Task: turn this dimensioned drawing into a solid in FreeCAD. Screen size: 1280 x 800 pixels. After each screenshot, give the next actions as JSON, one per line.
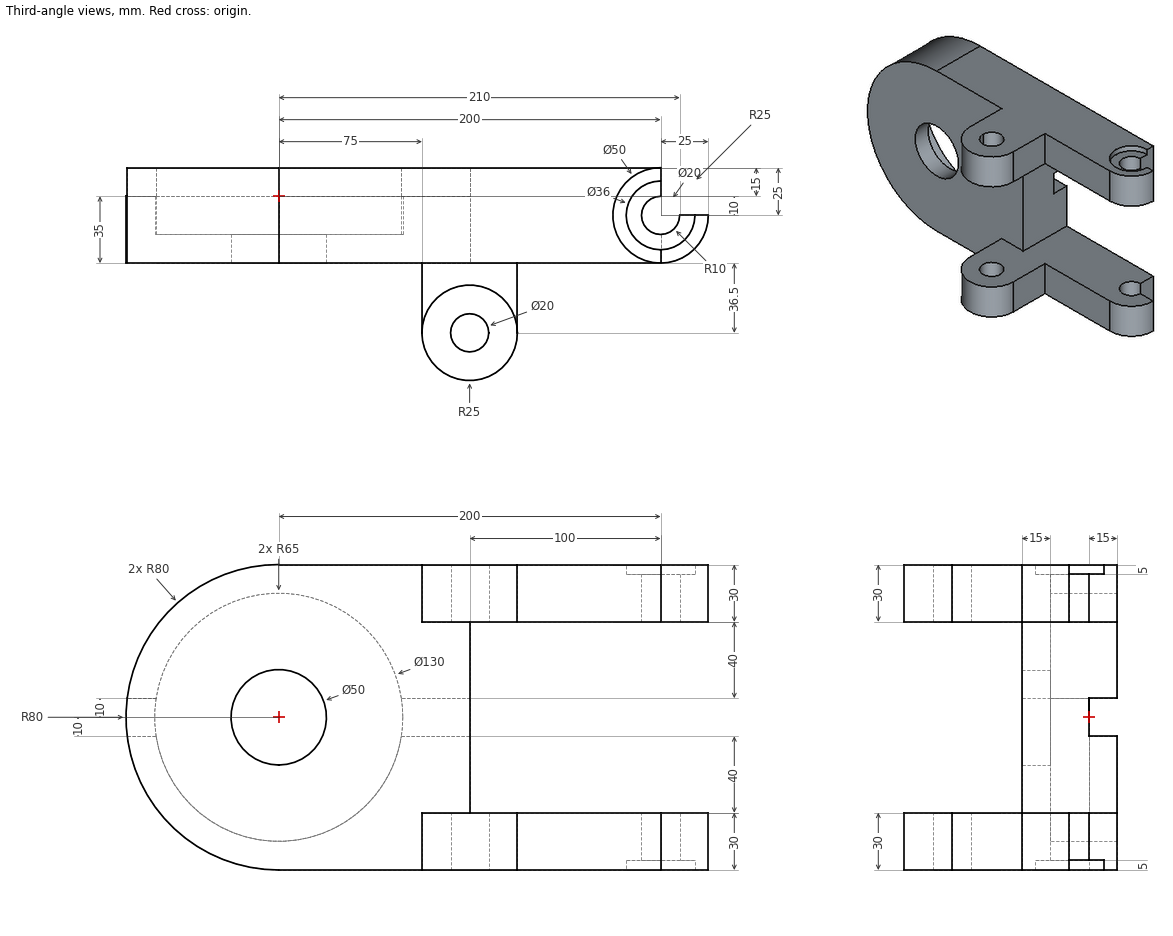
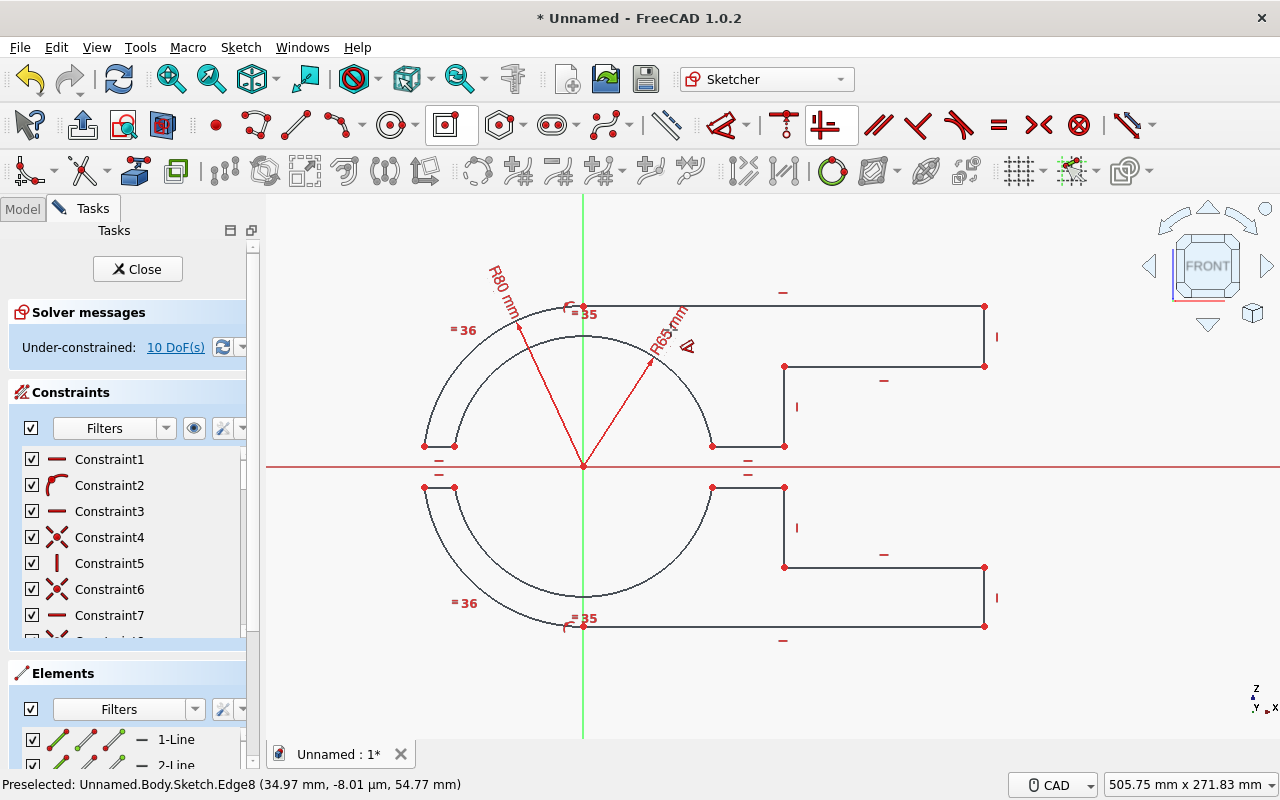
{"action": "left_click", "coordinate": [984, 324]}
{"action": "left_click", "coordinate": [1018, 337]}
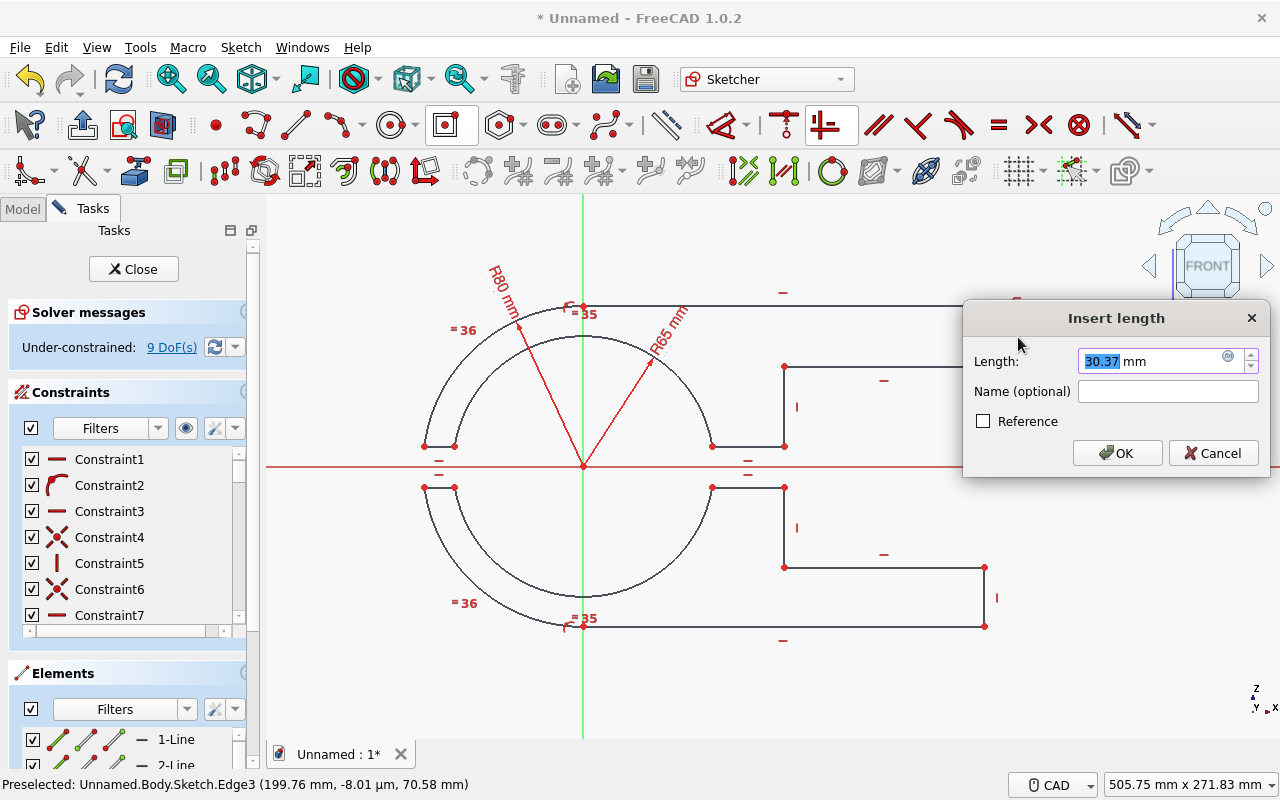
{"action": "type", "text": "30"}
{"action": "key", "text": "Return"}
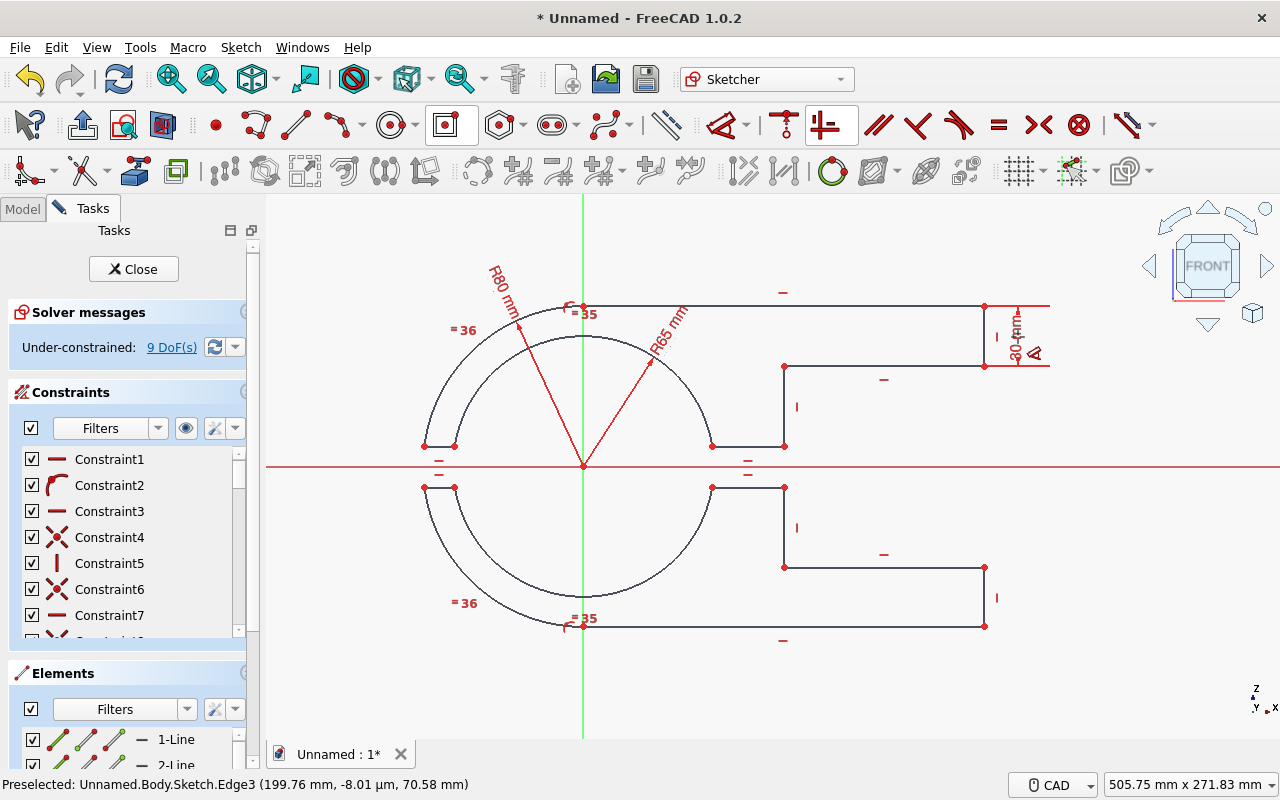
{"action": "left_click", "coordinate": [784, 390]}
{"action": "left_click", "coordinate": [818, 407]}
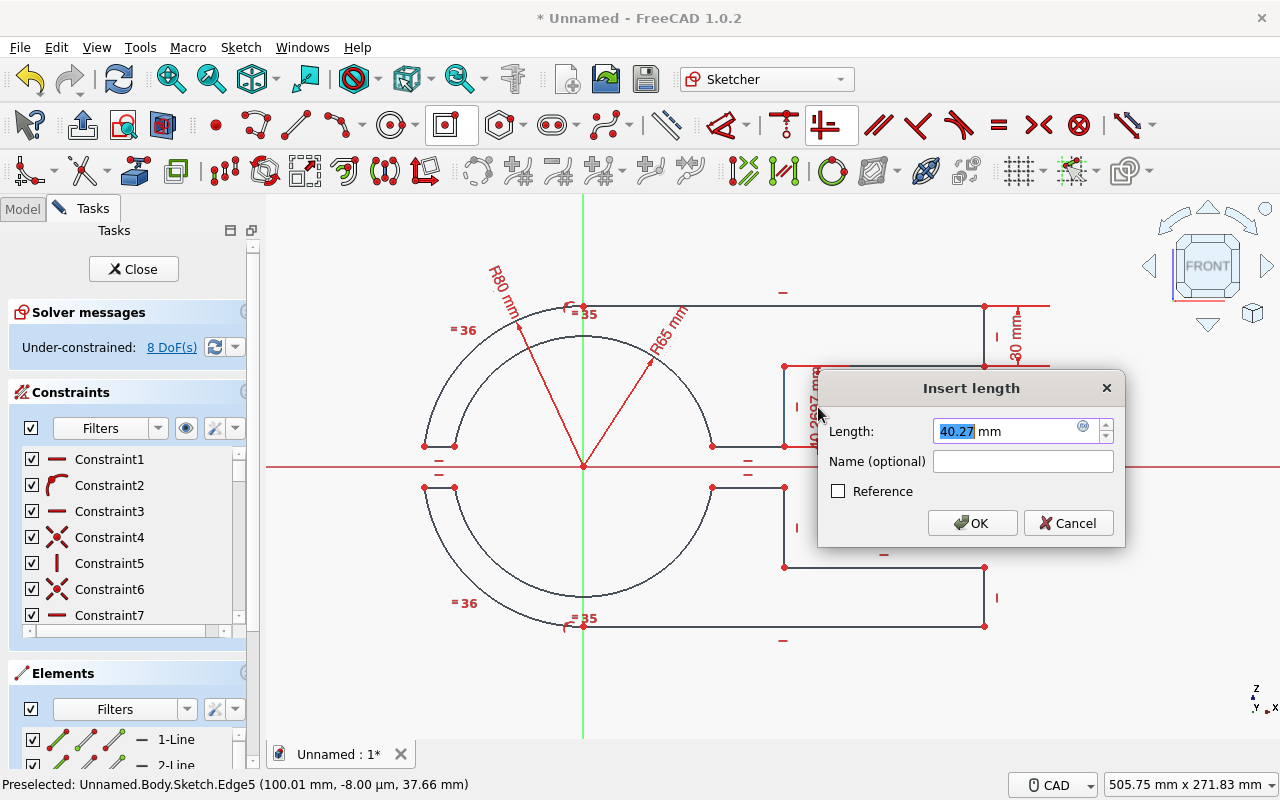
{"action": "type", "text": "40"}
{"action": "key", "text": "Return"}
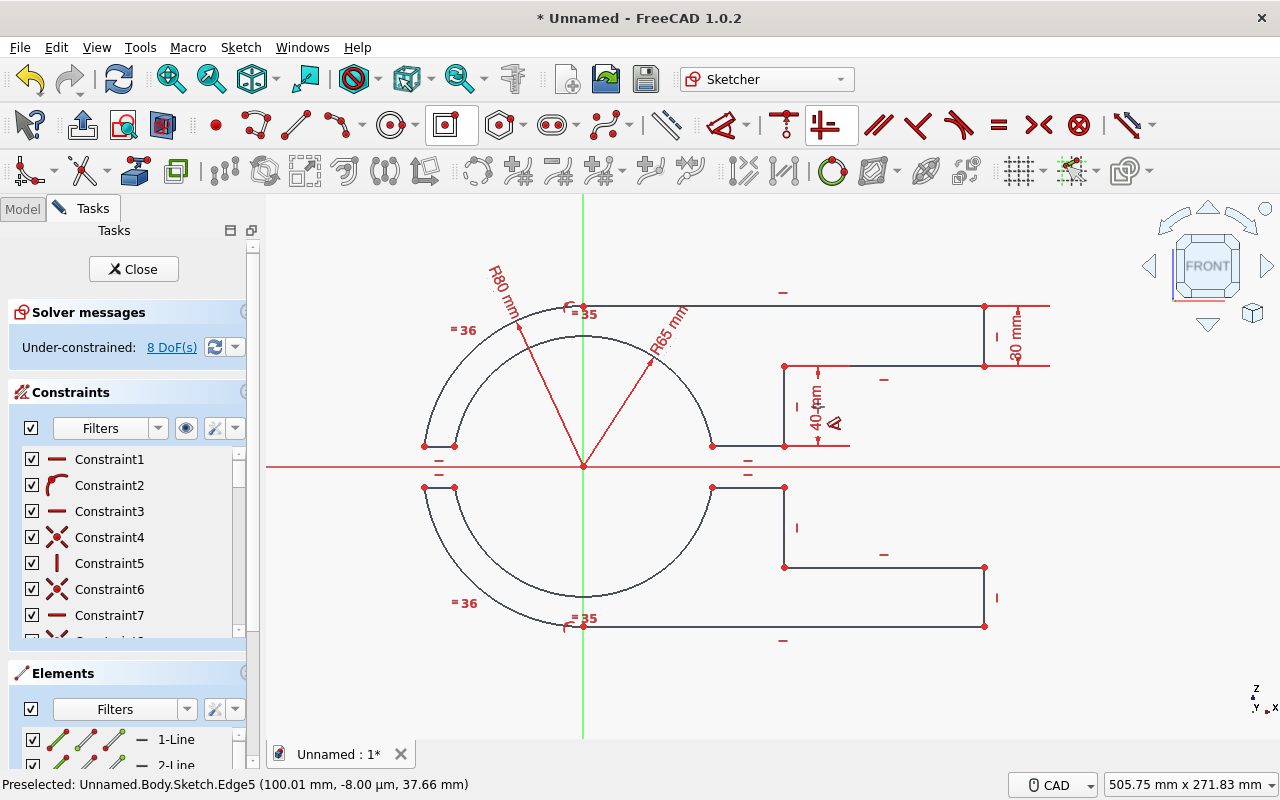
{"action": "left_click", "coordinate": [784, 512]}
{"action": "left_click", "coordinate": [818, 528]}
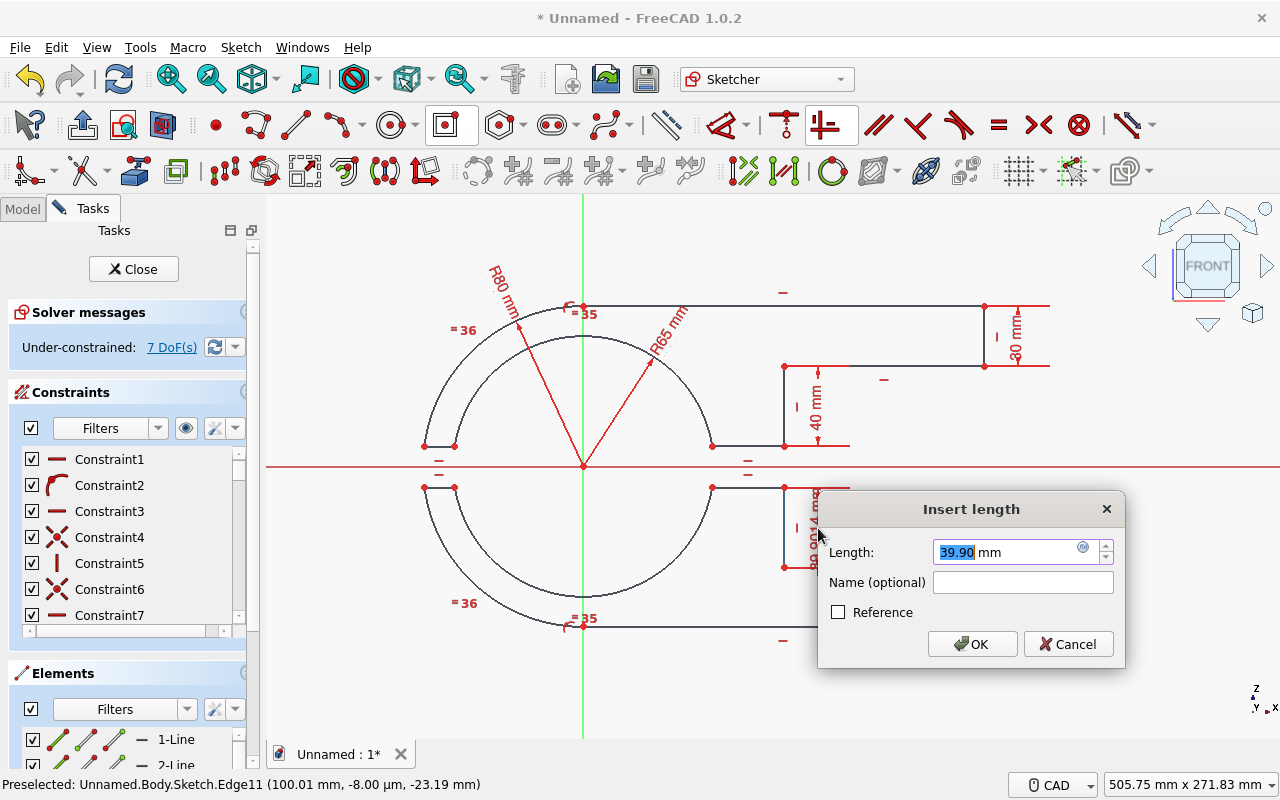
{"action": "type", "text": "40"}
{"action": "key", "text": "Return"}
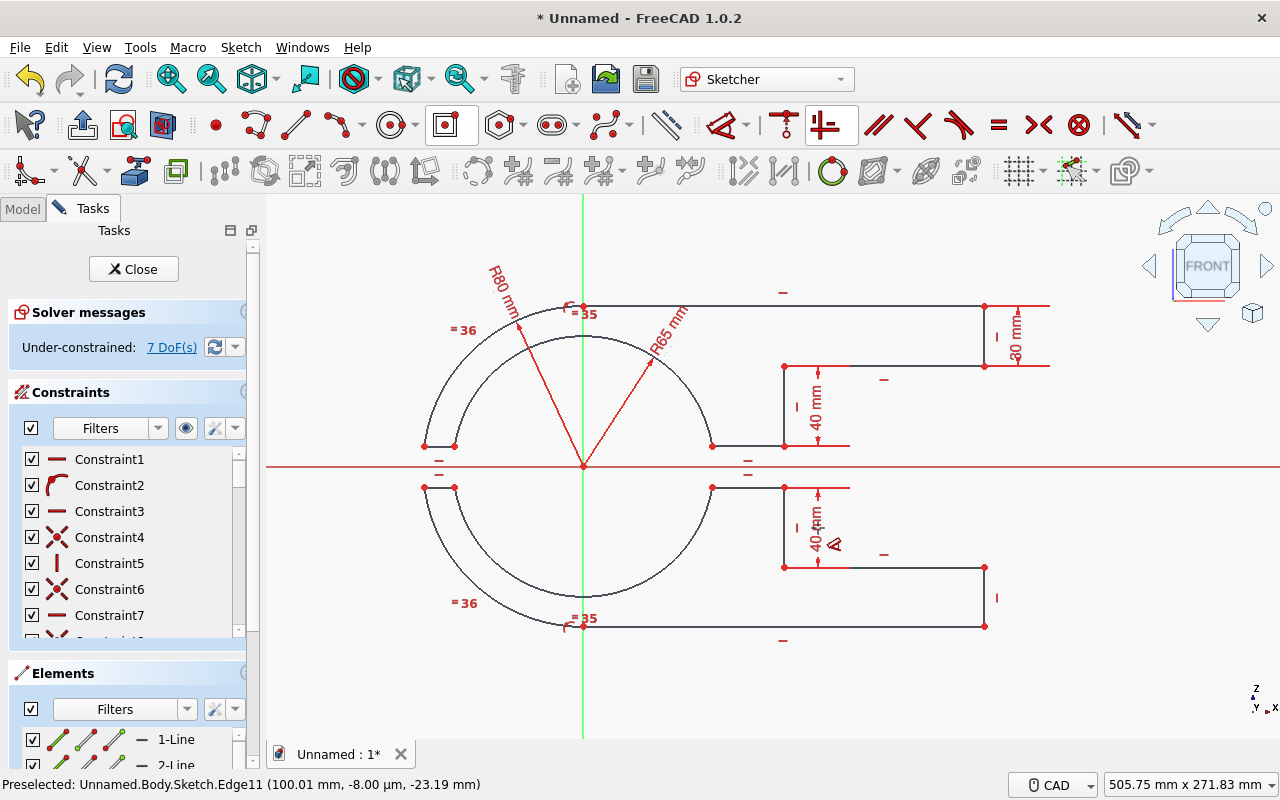
{"action": "left_click", "coordinate": [984, 586]}
{"action": "left_click", "coordinate": [1018, 597]}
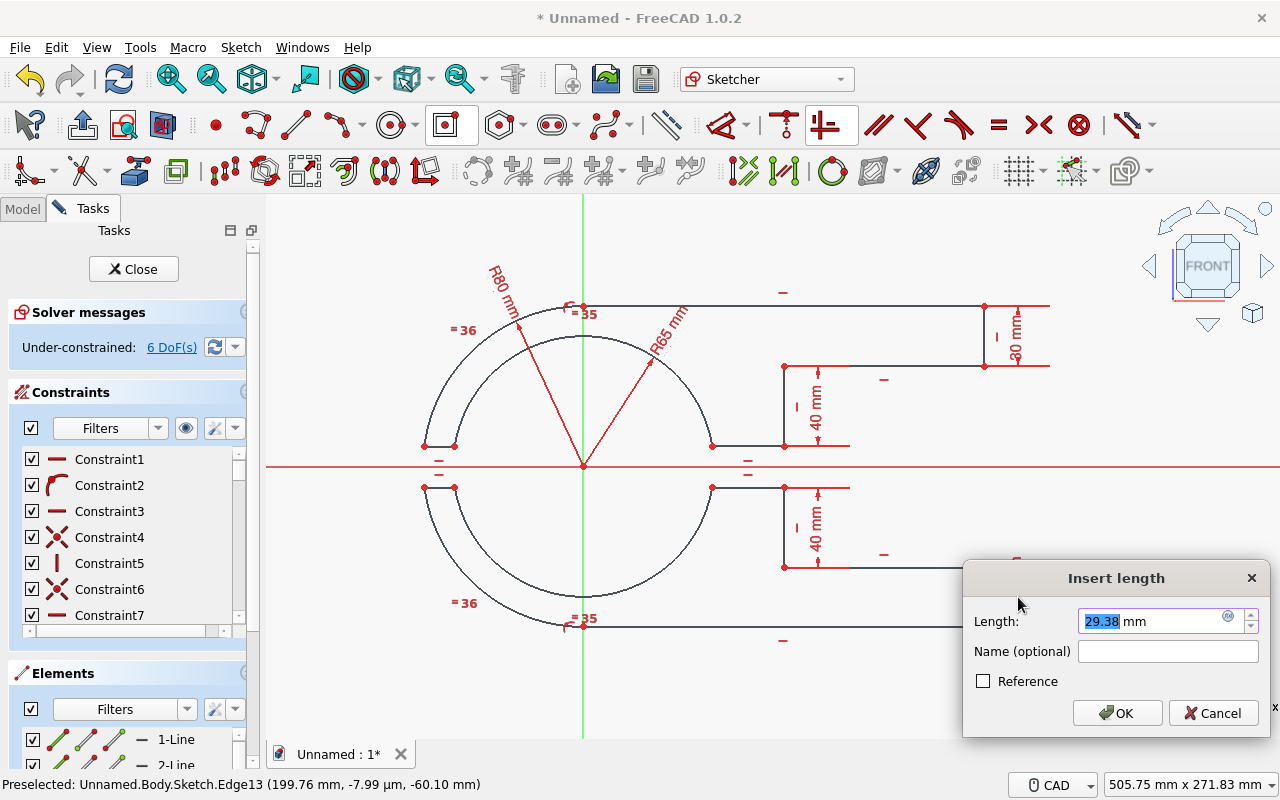
{"action": "type", "text": "30"}
{"action": "key", "text": "Return"}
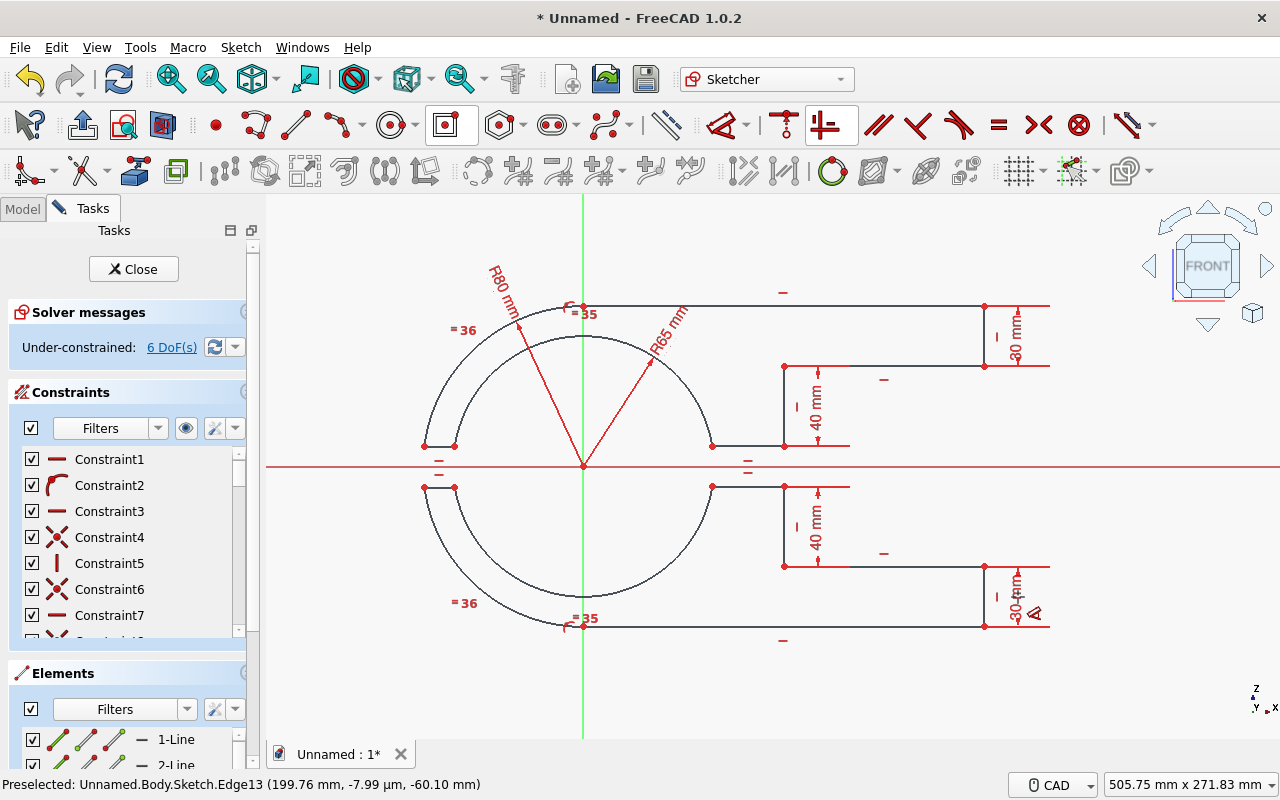
{"action": "left_click", "coordinate": [704, 306]}
{"action": "left_click", "coordinate": [784, 272]}